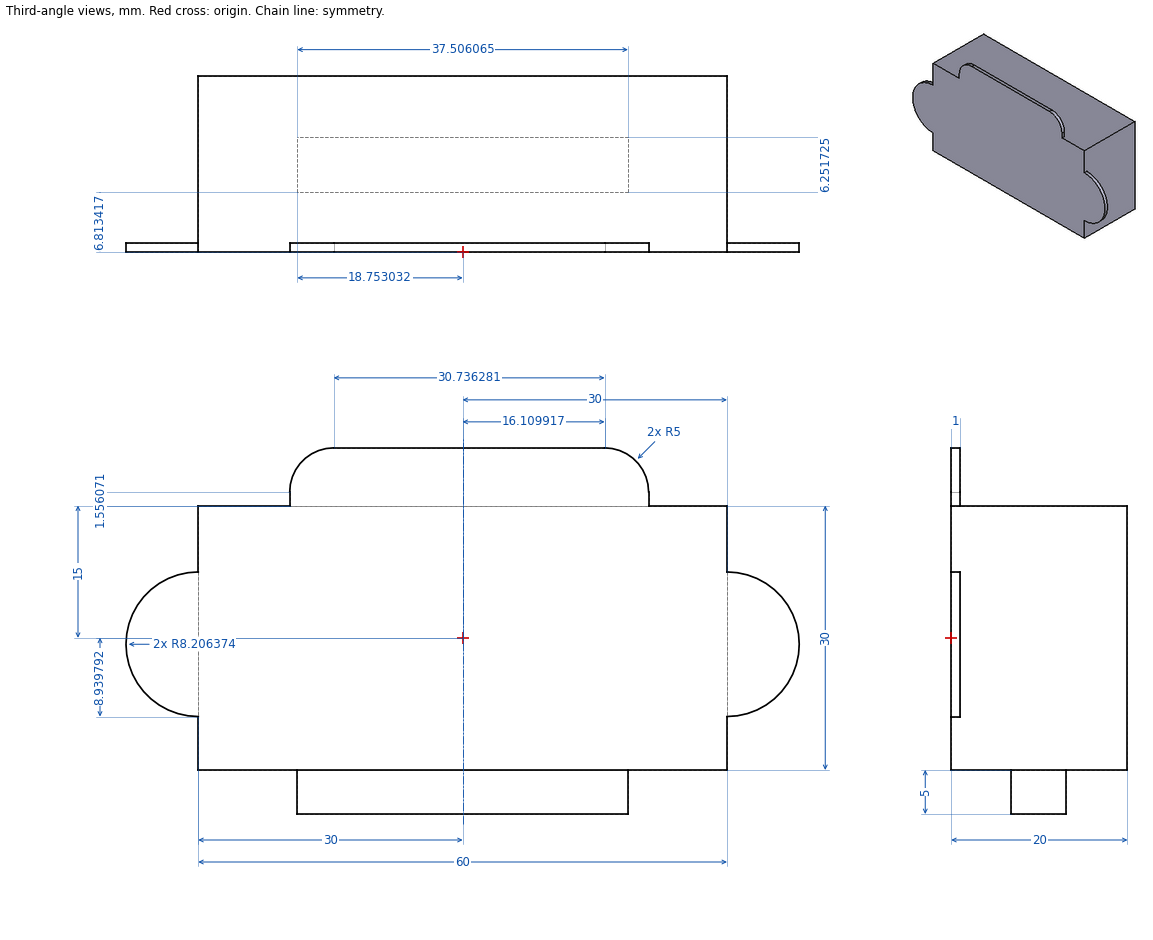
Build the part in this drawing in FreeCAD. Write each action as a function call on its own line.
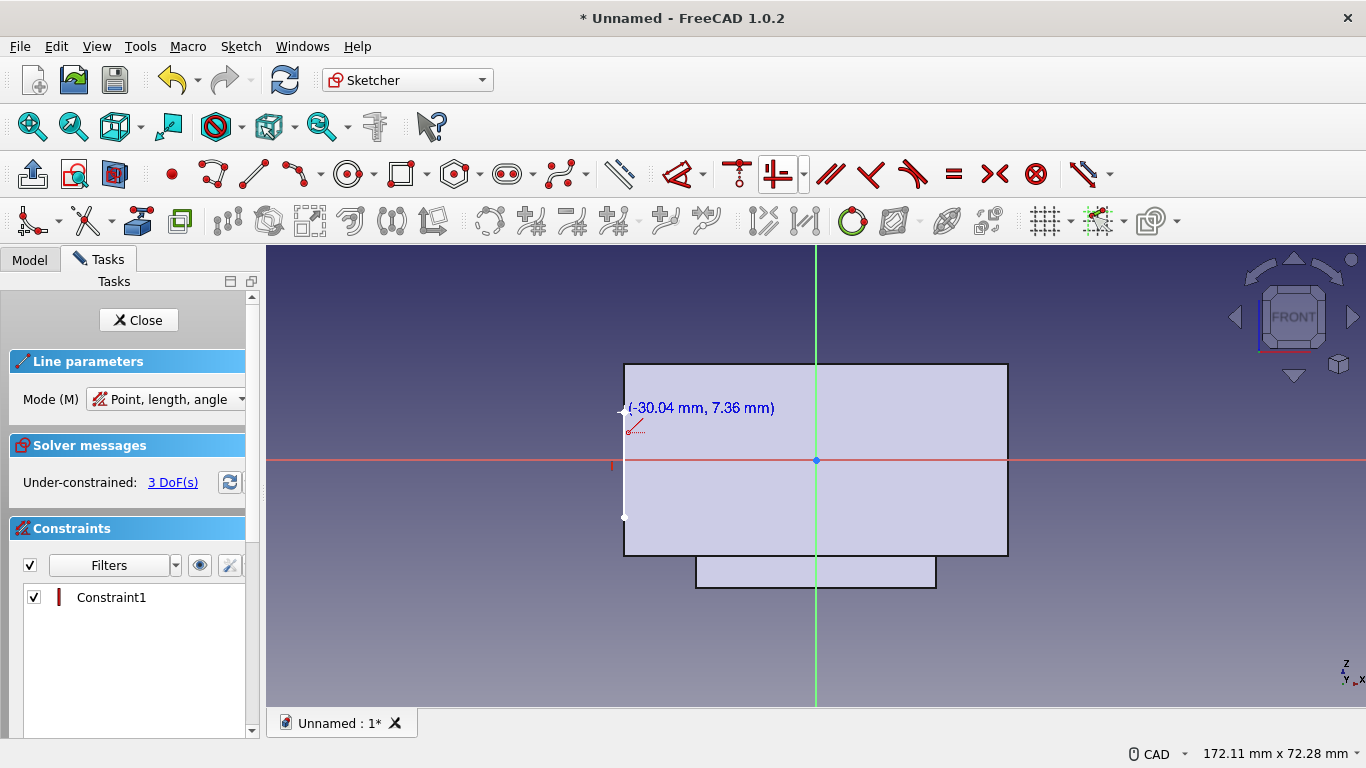
key(g)
key(3)
key(a)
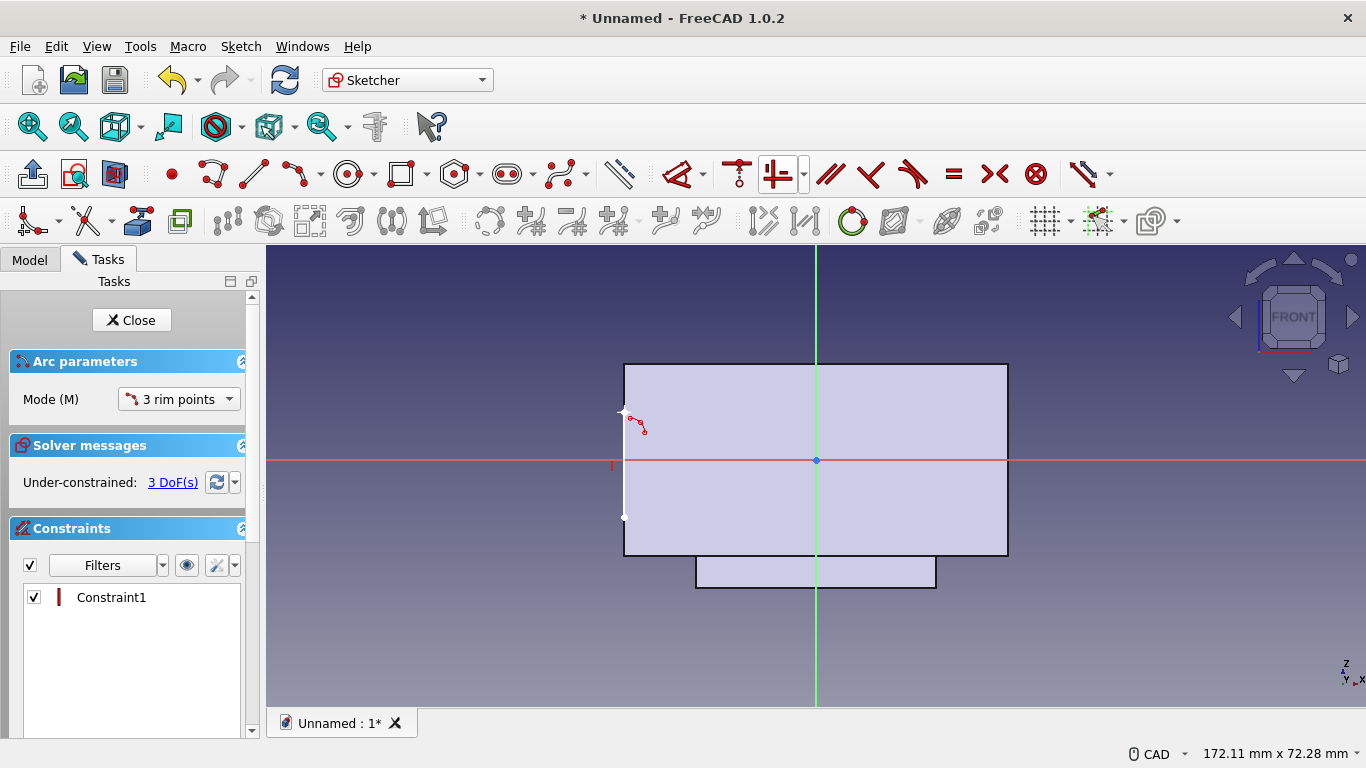
click(624, 413)
click(624, 518)
click(574, 481)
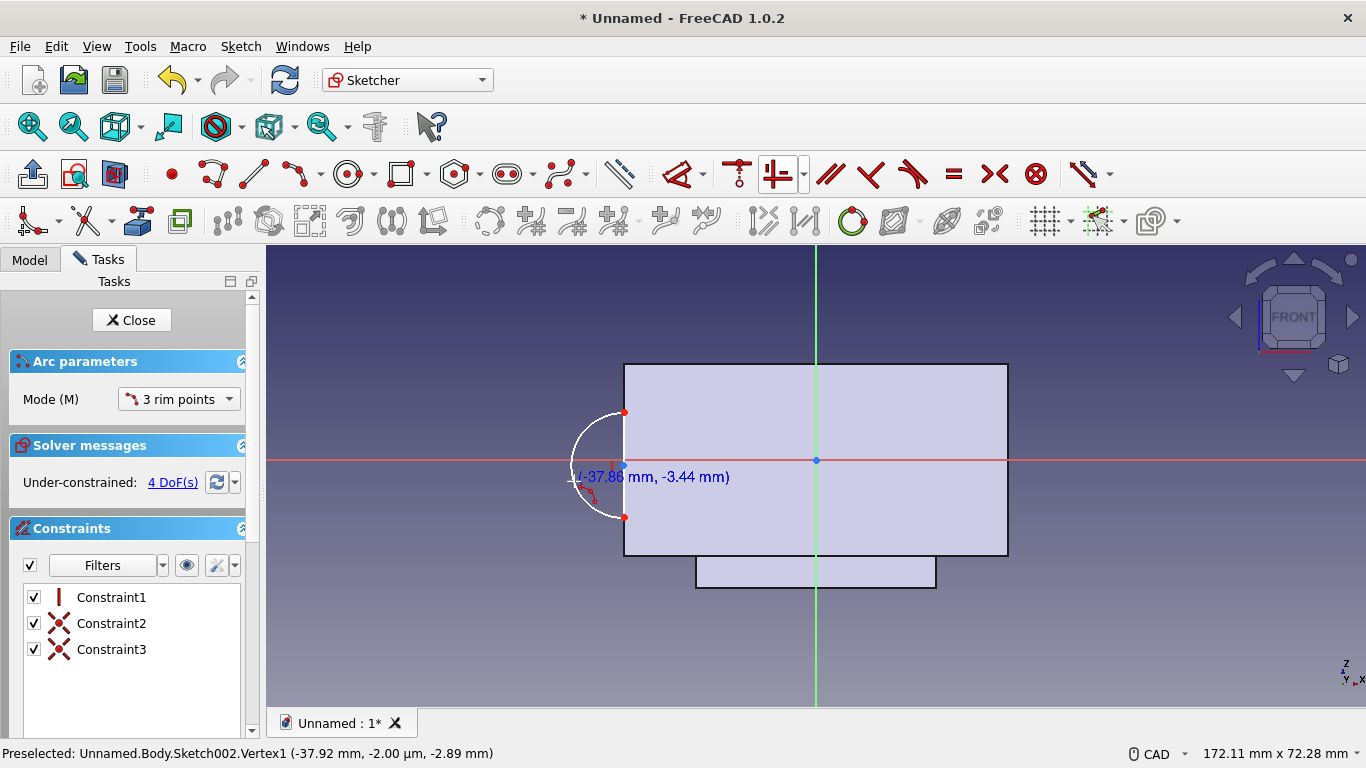
key(g)
key(l)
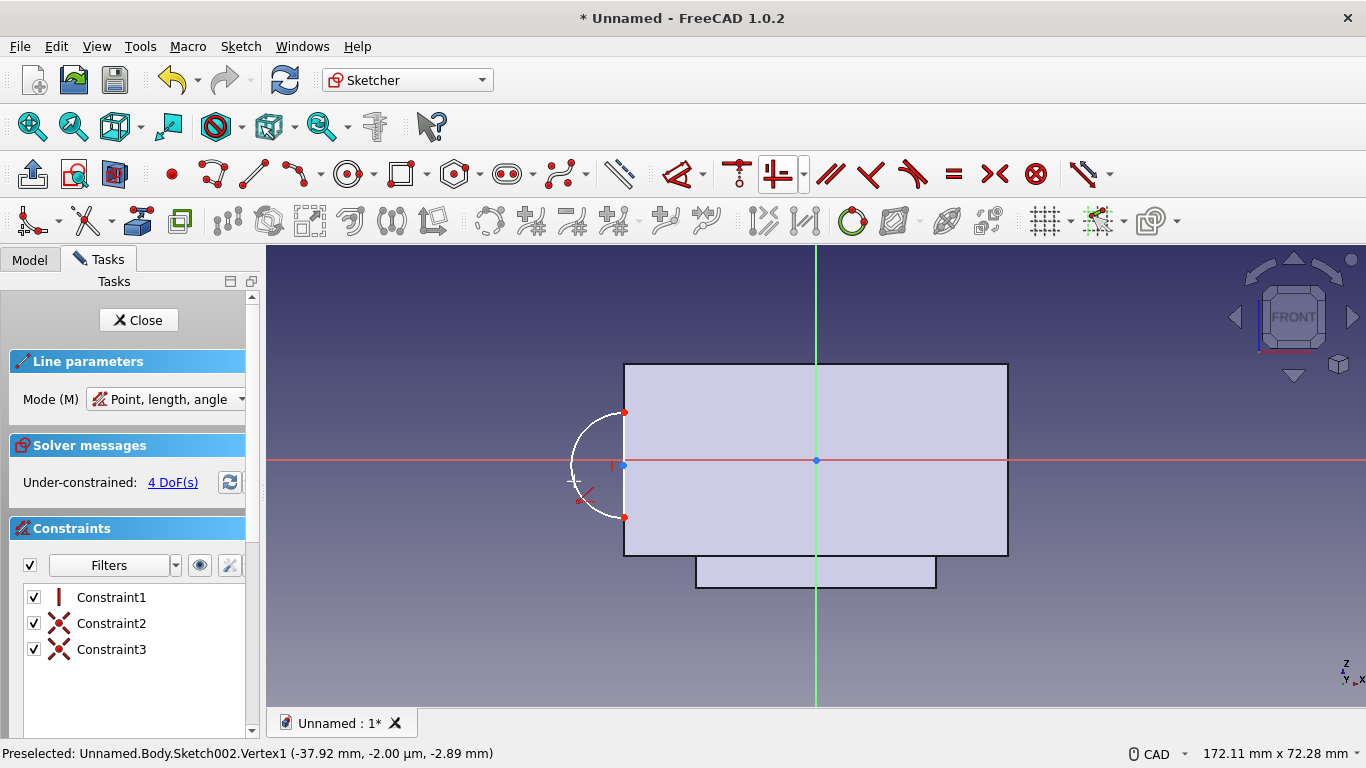
click(1008, 412)
click(1008, 517)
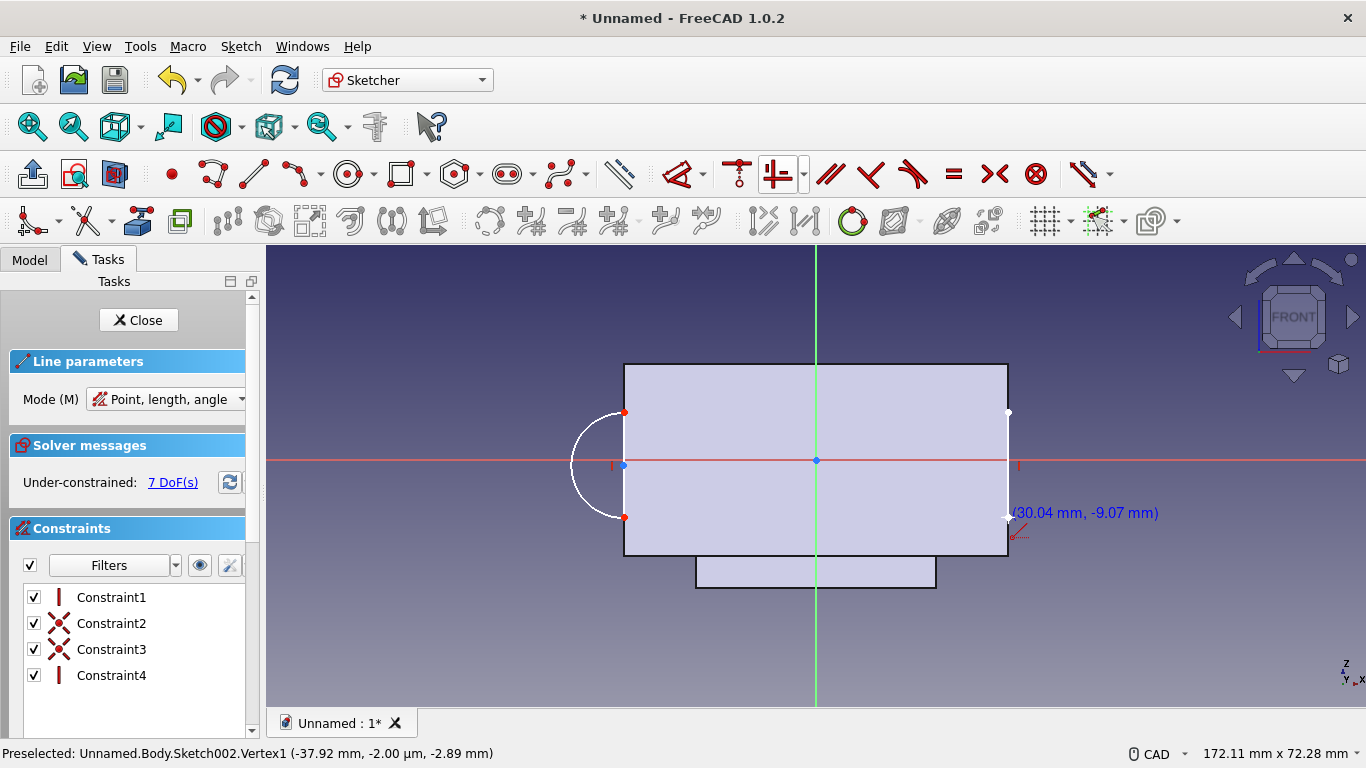
click(294, 174)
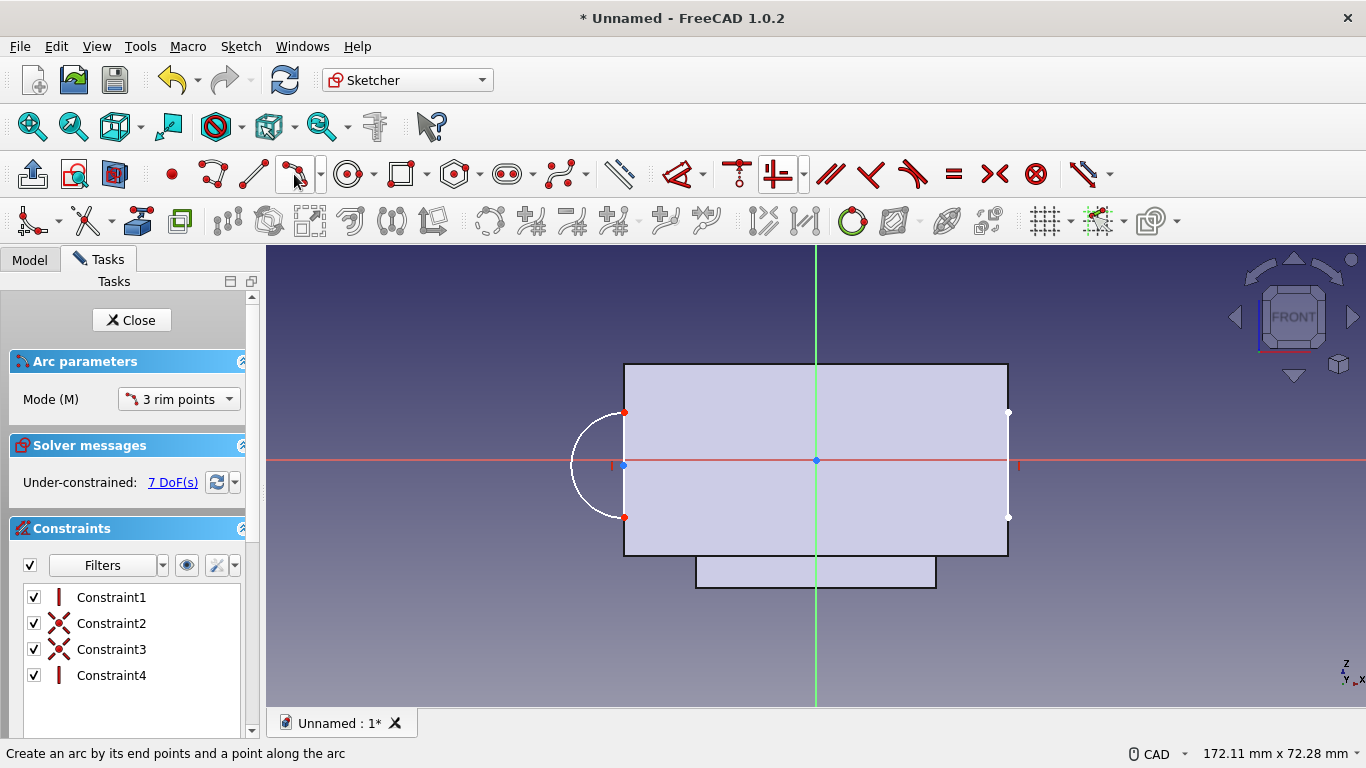
click(1008, 518)
click(1008, 413)
click(1058, 481)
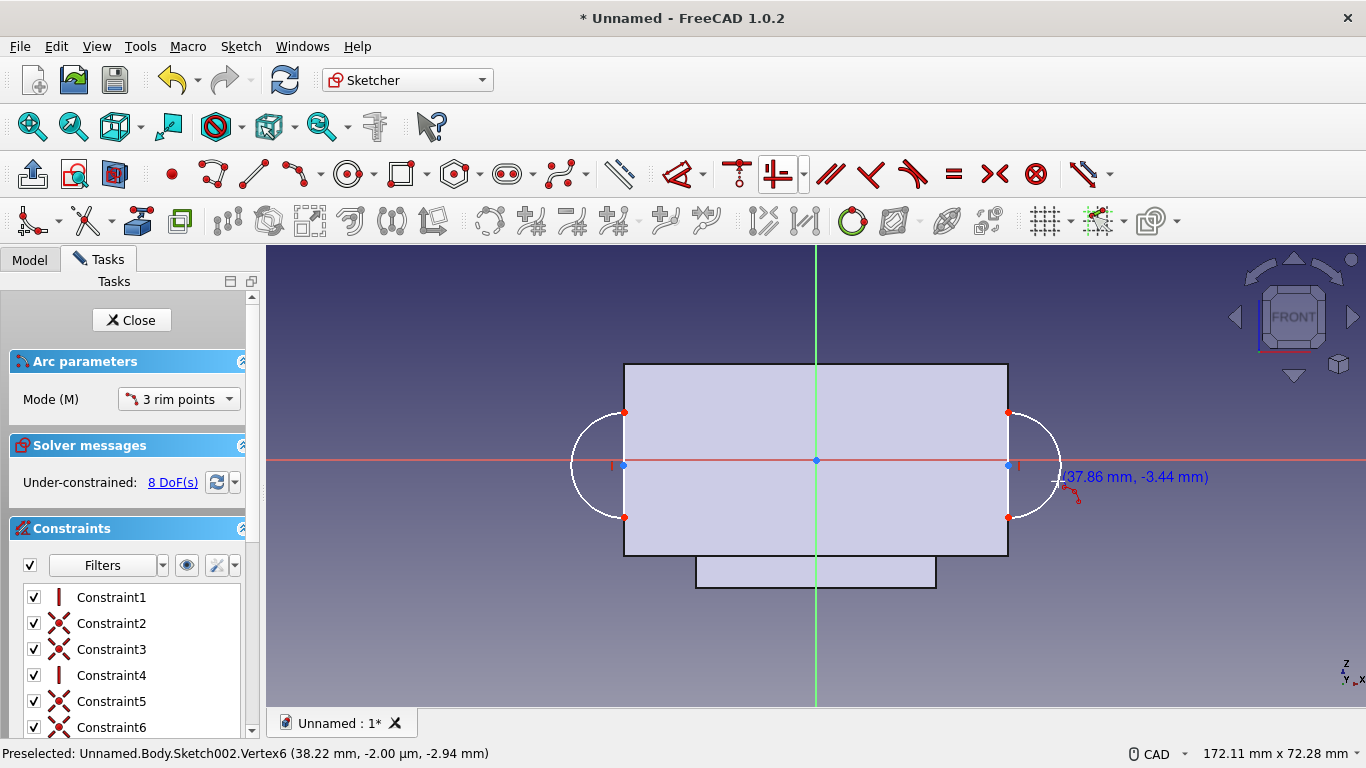
key(g)
key(l)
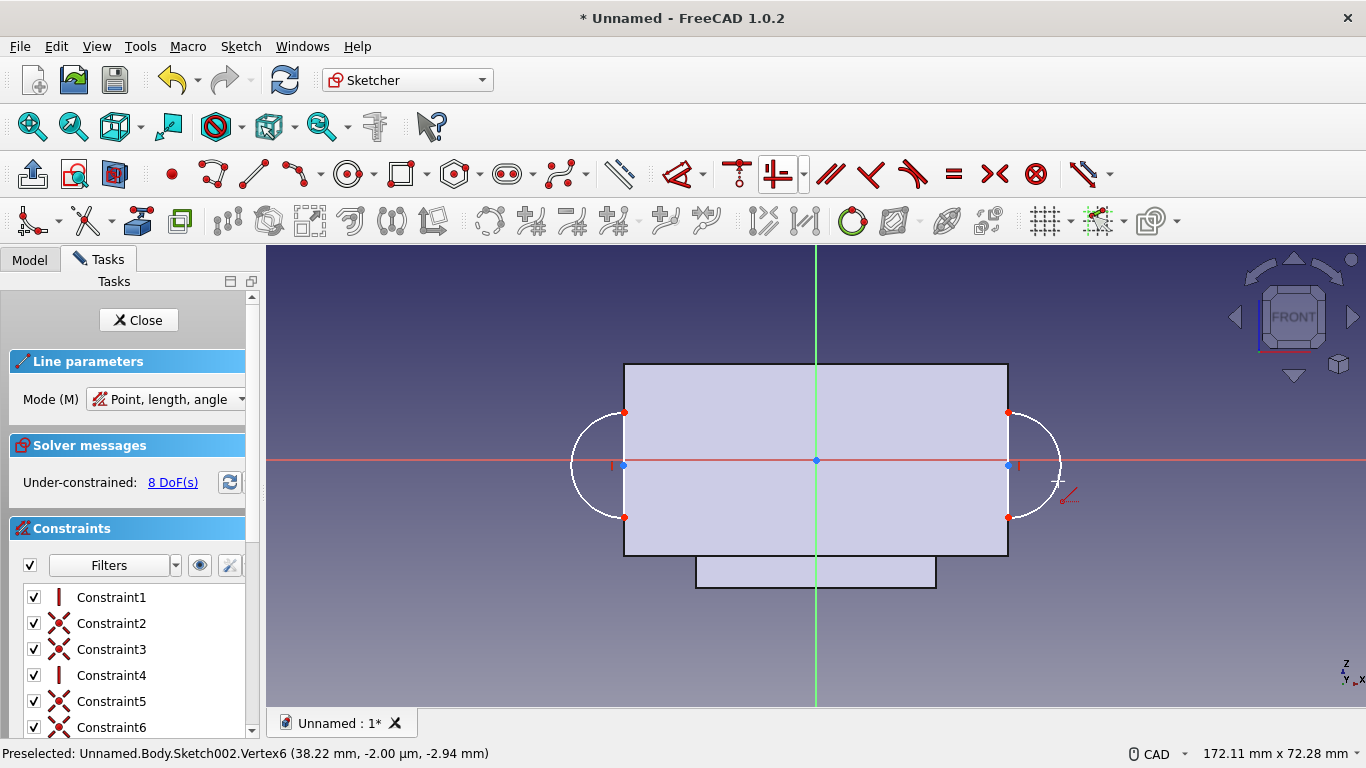
click(919, 322)
click(723, 322)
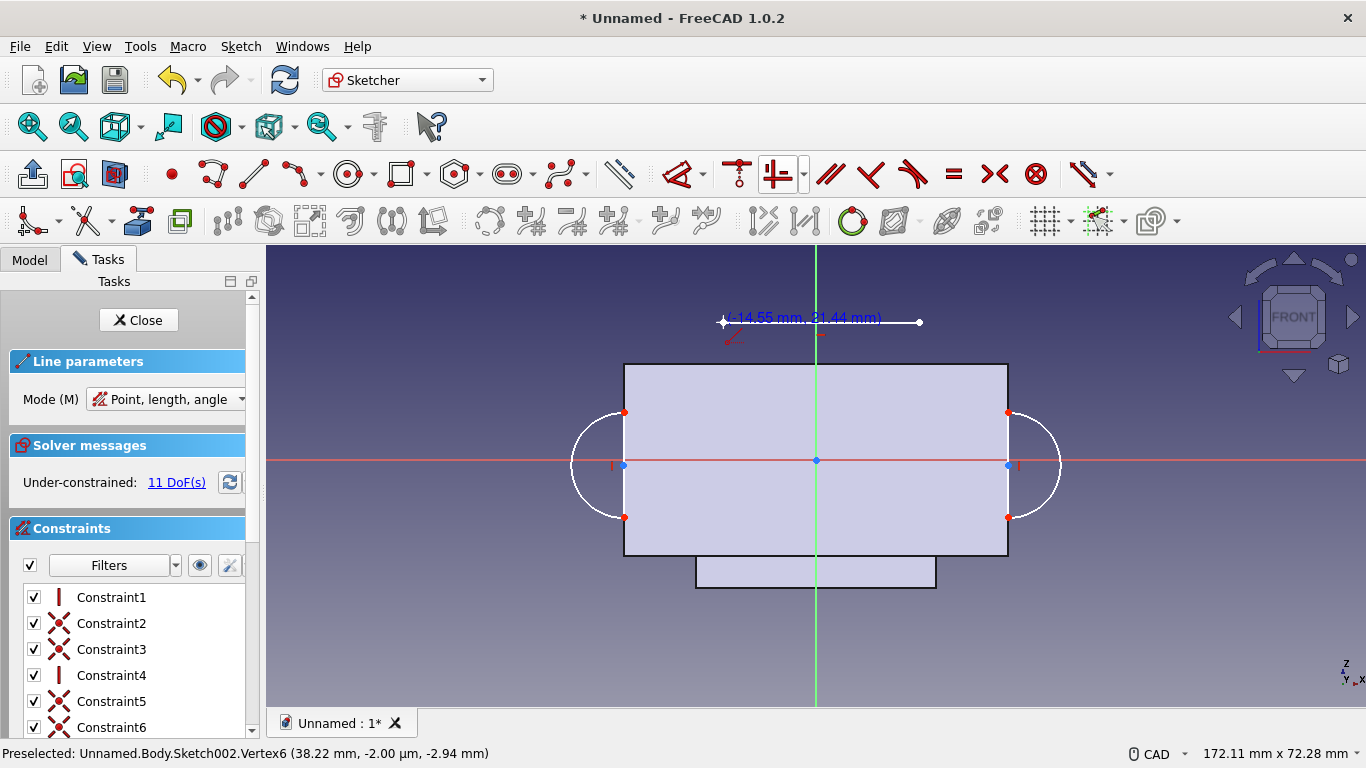
key(g)
key(m)